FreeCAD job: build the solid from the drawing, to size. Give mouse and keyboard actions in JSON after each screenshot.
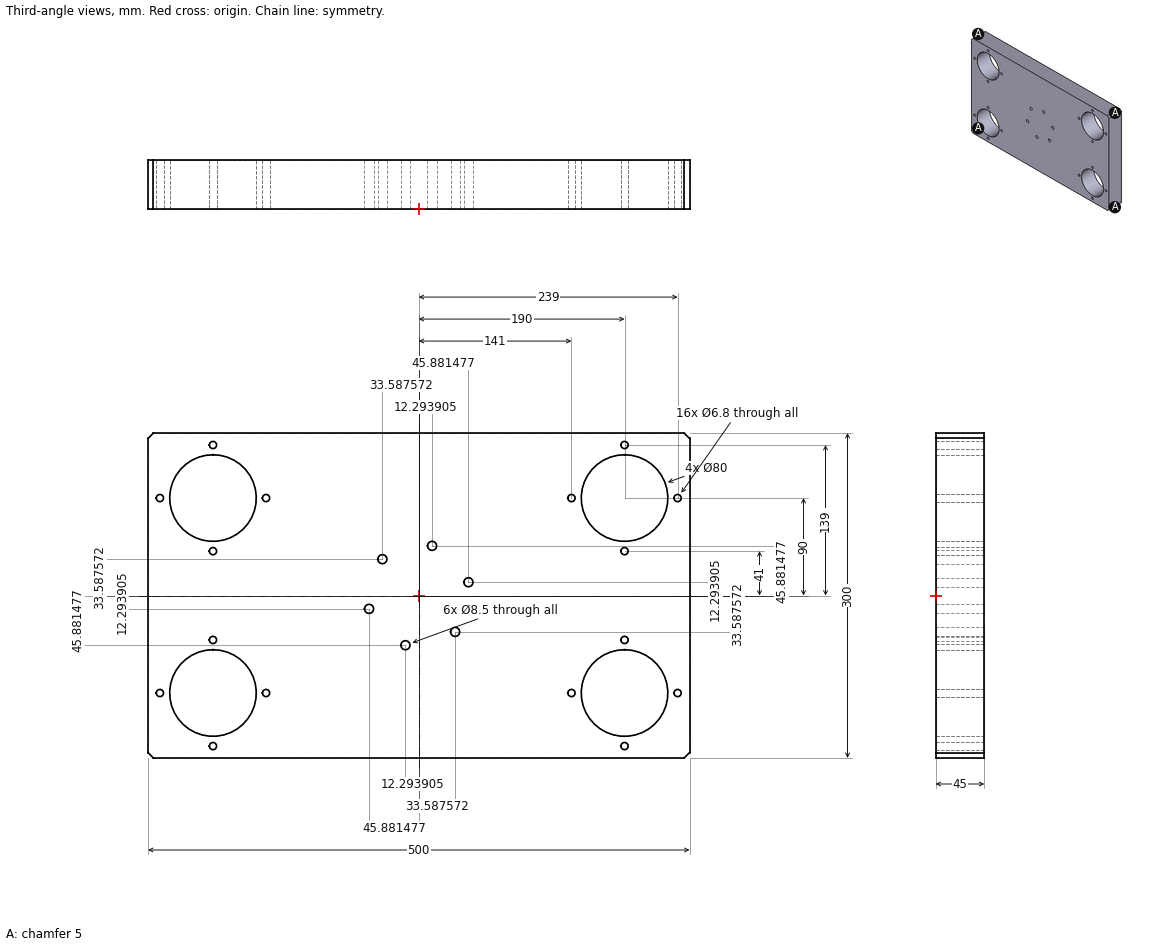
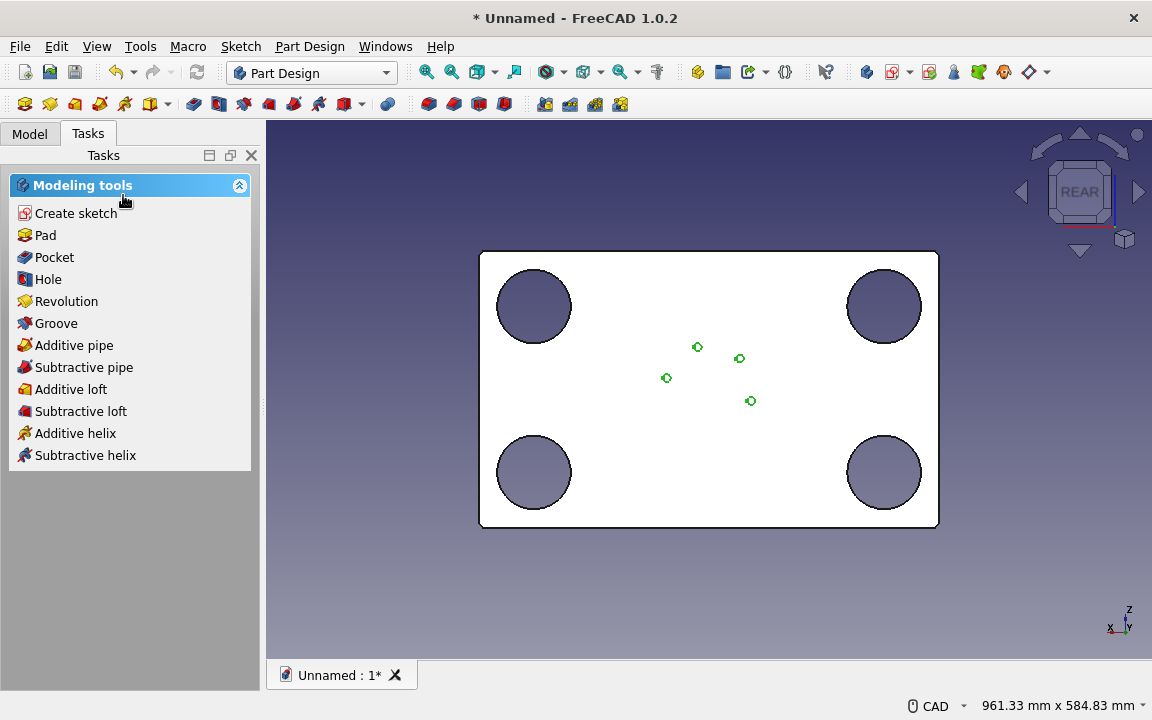
{"action": "left_click", "coordinate": [219, 104]}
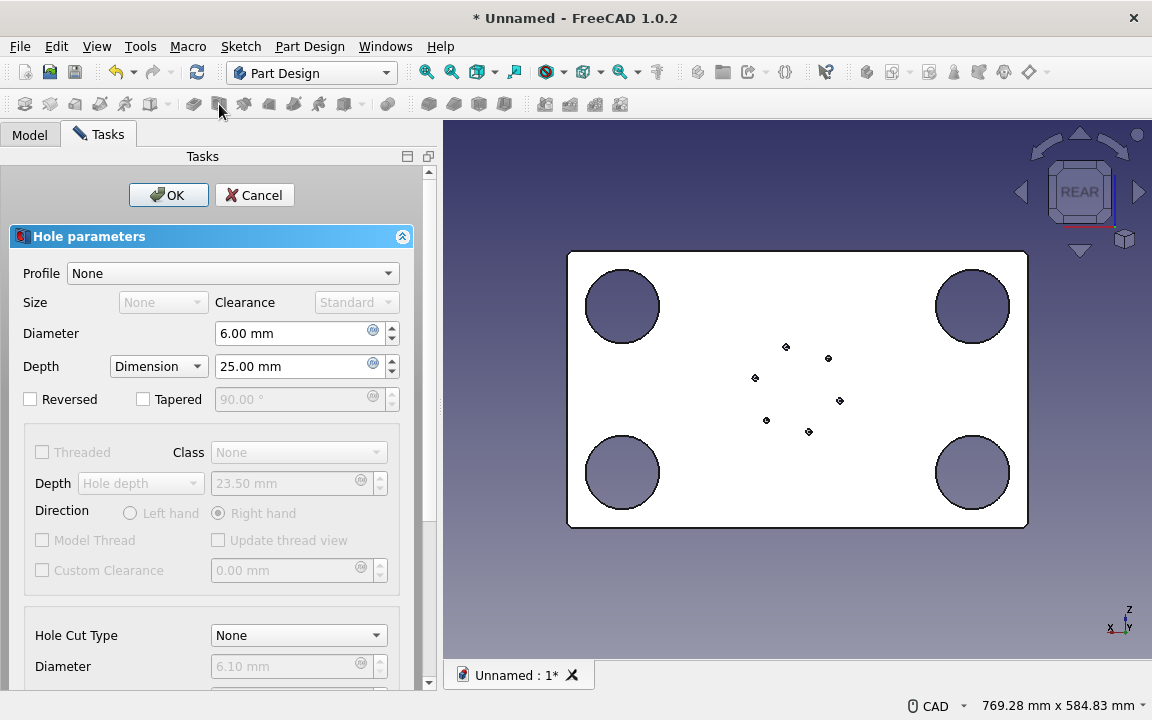
{"action": "triple_click", "coordinate": [300, 334]}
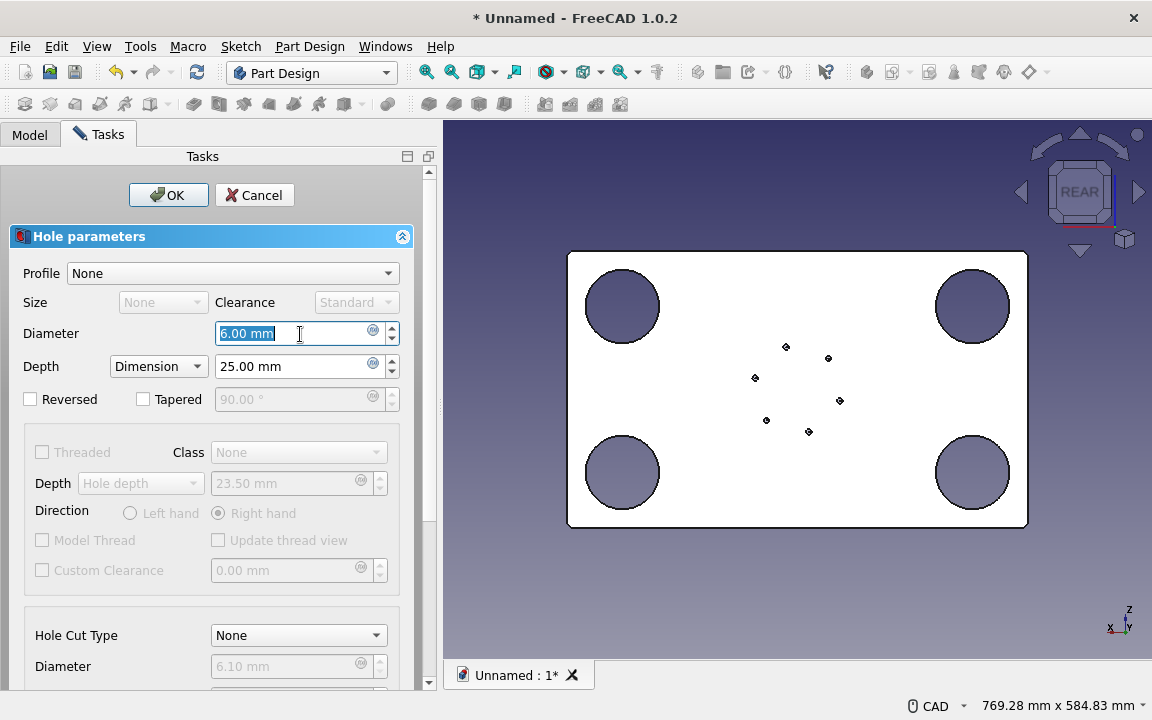
{"action": "type", "text": "8.5"}
{"action": "key", "text": "Tab"}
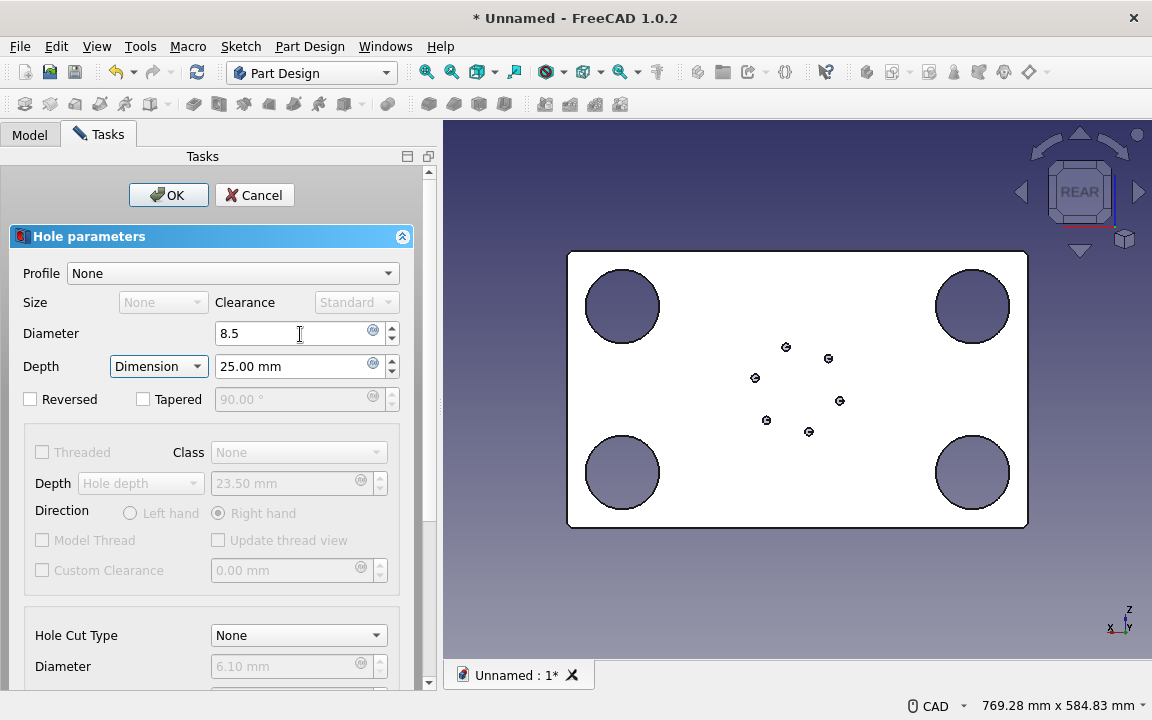
{"action": "left_click", "coordinate": [160, 366]}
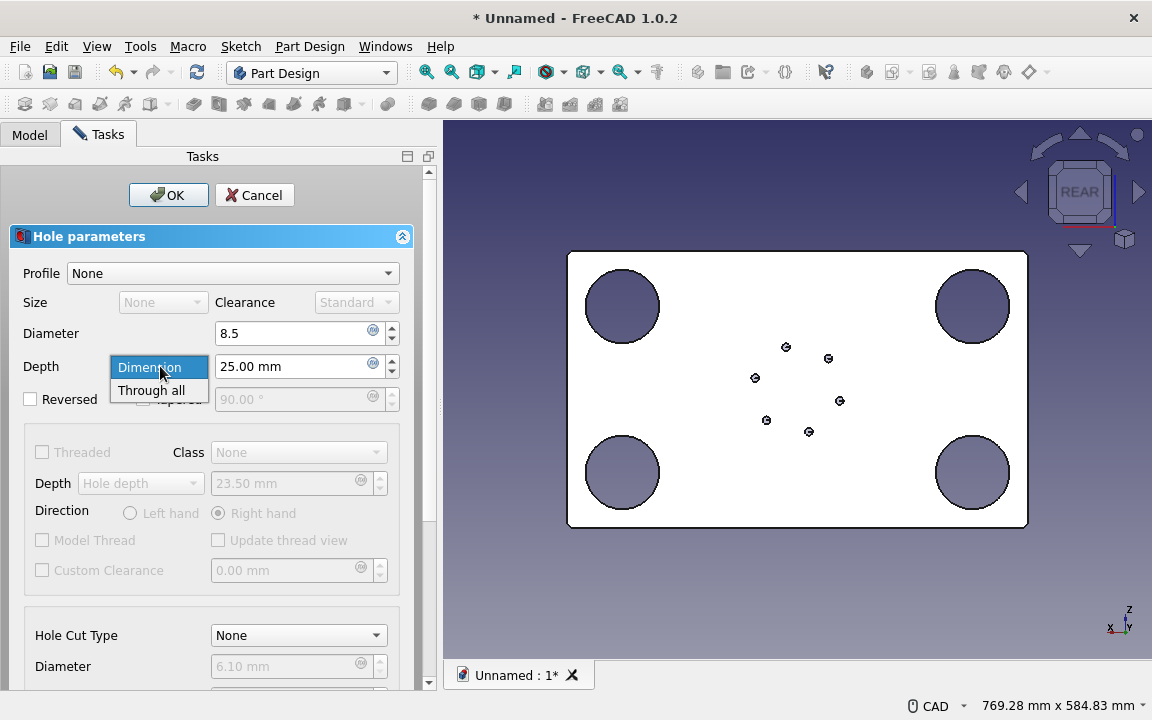
{"action": "left_click", "coordinate": [158, 390]}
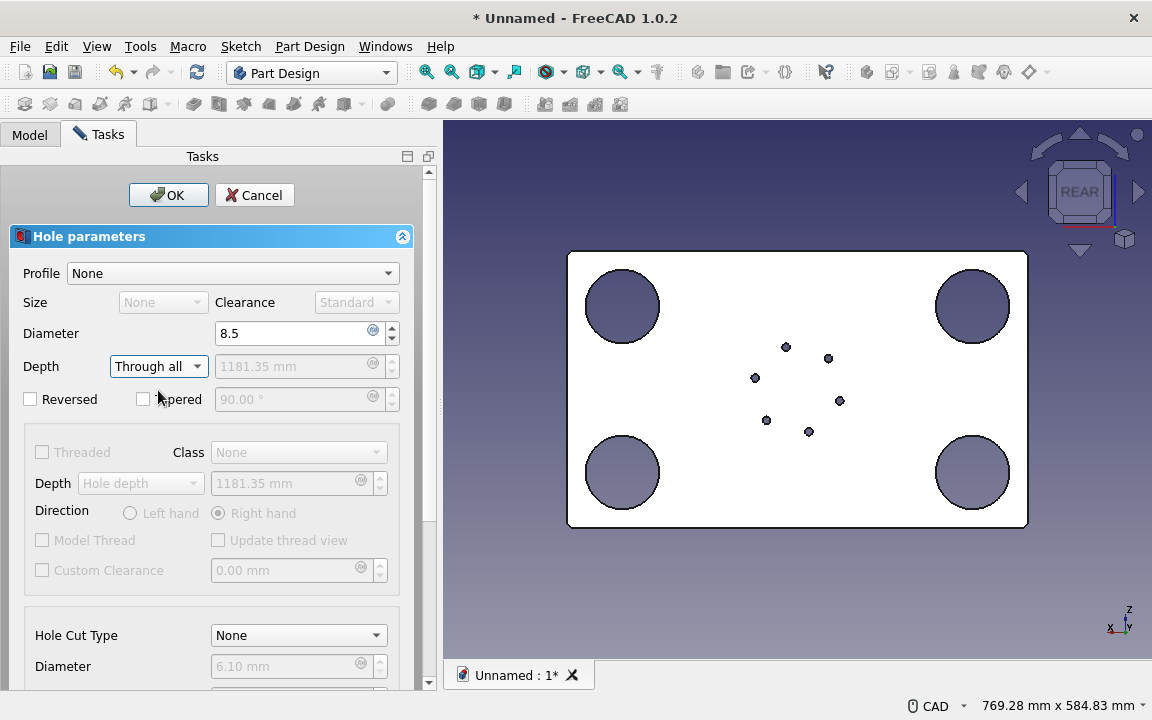
{"action": "left_click", "coordinate": [169, 195]}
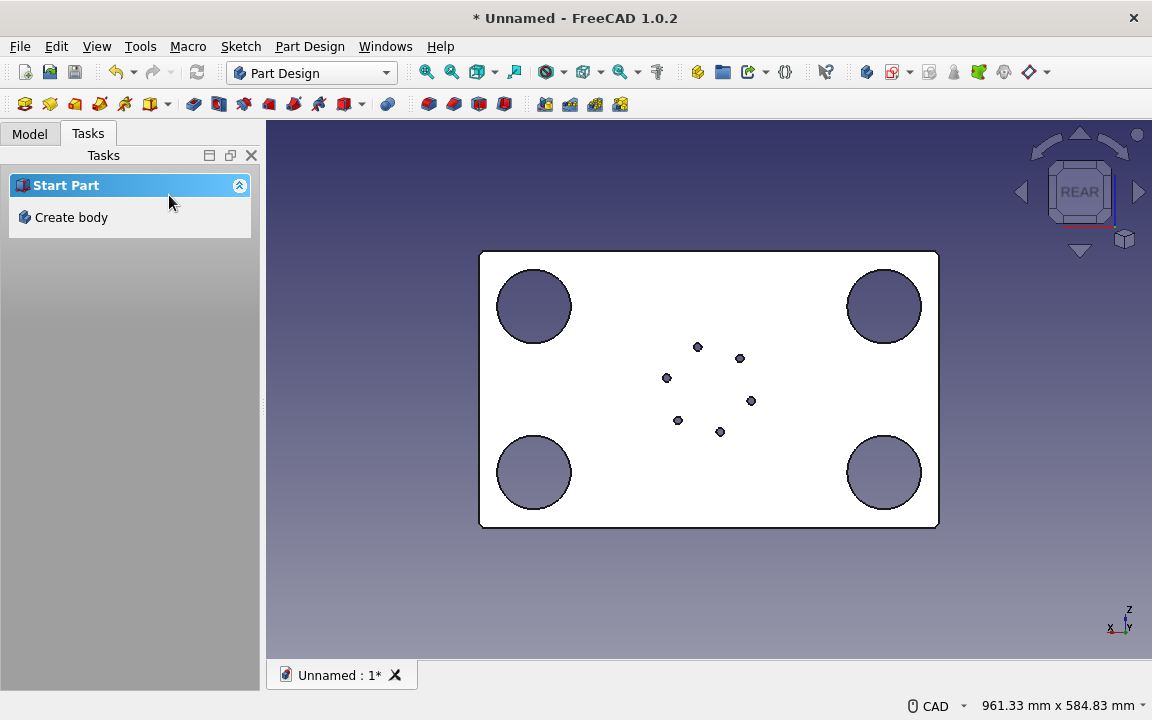
{"action": "left_click", "coordinate": [643, 310]}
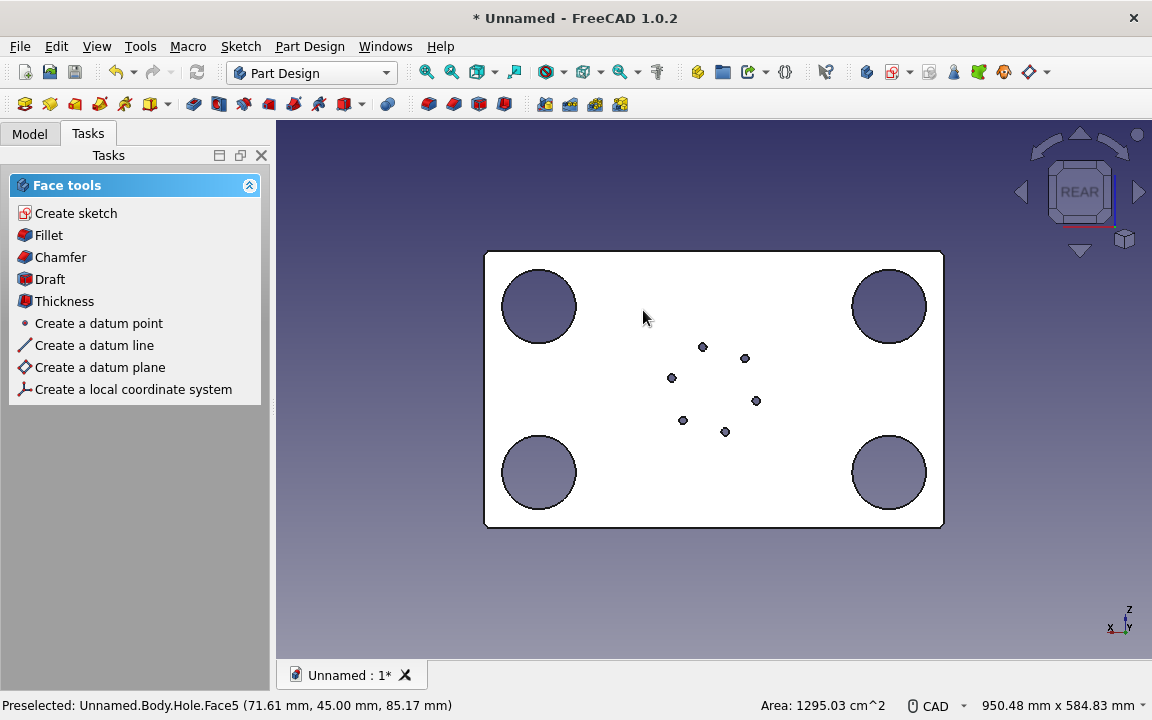
{"action": "left_click", "coordinate": [892, 72]}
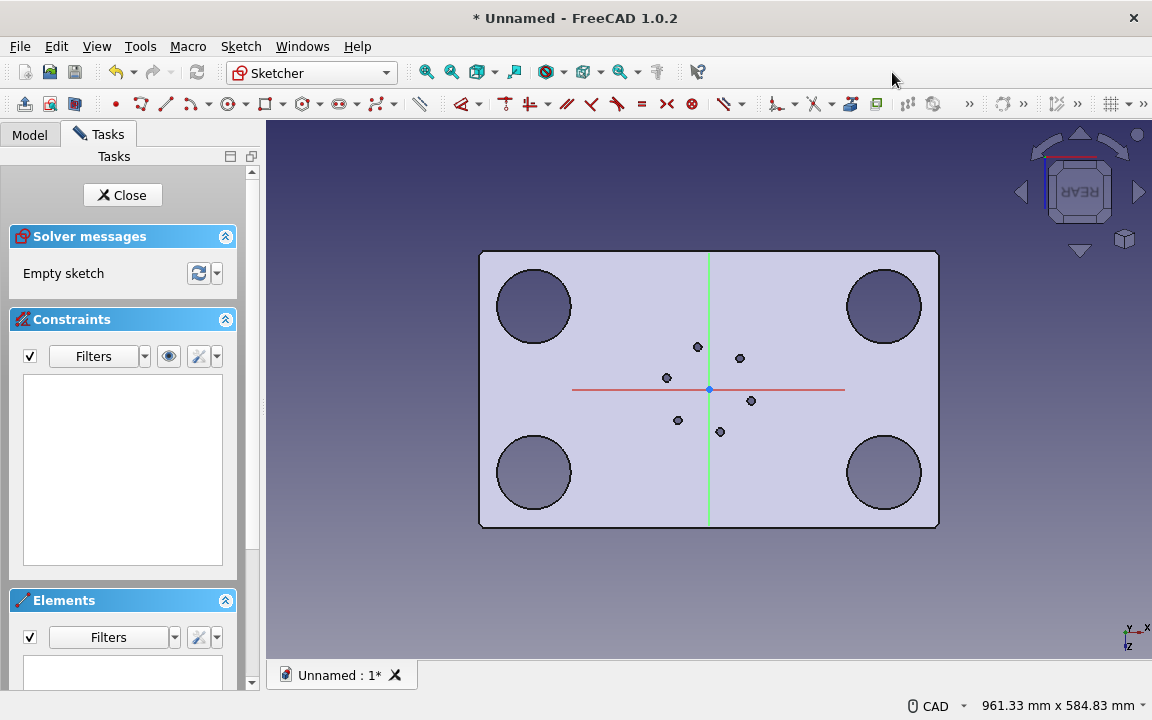
{"action": "left_click", "coordinate": [228, 104]}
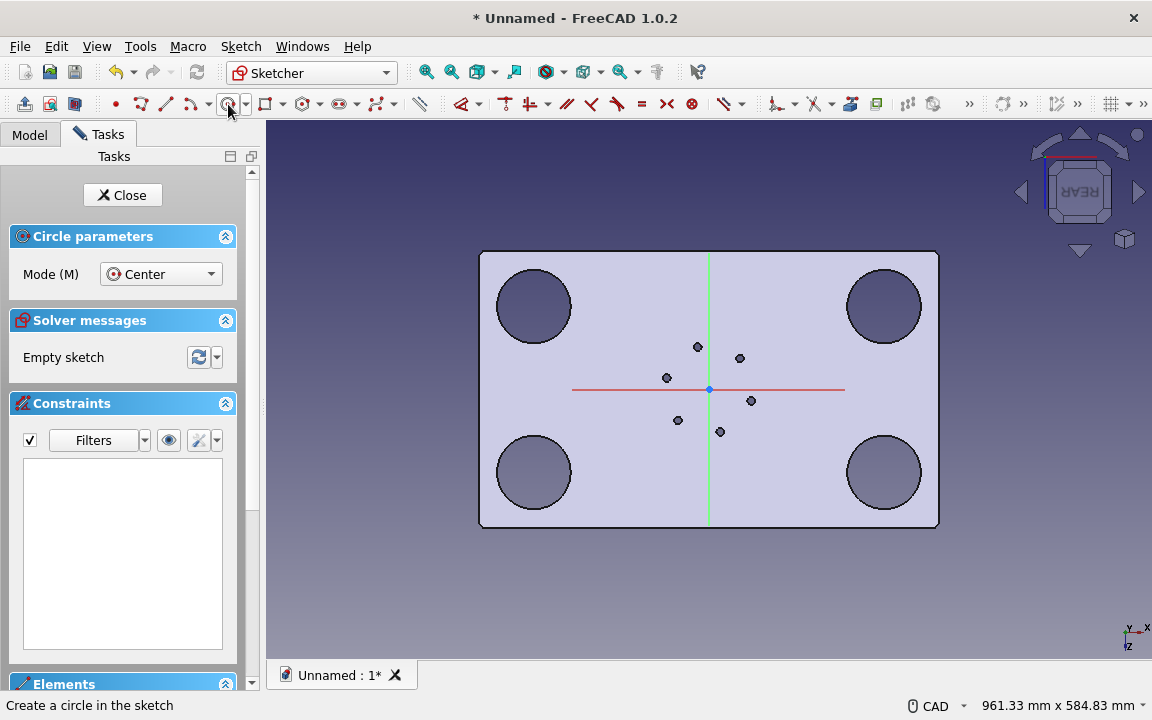
{"action": "scroll", "coordinate": [929, 472], "scroll_direction": "up", "scroll_amount": 10}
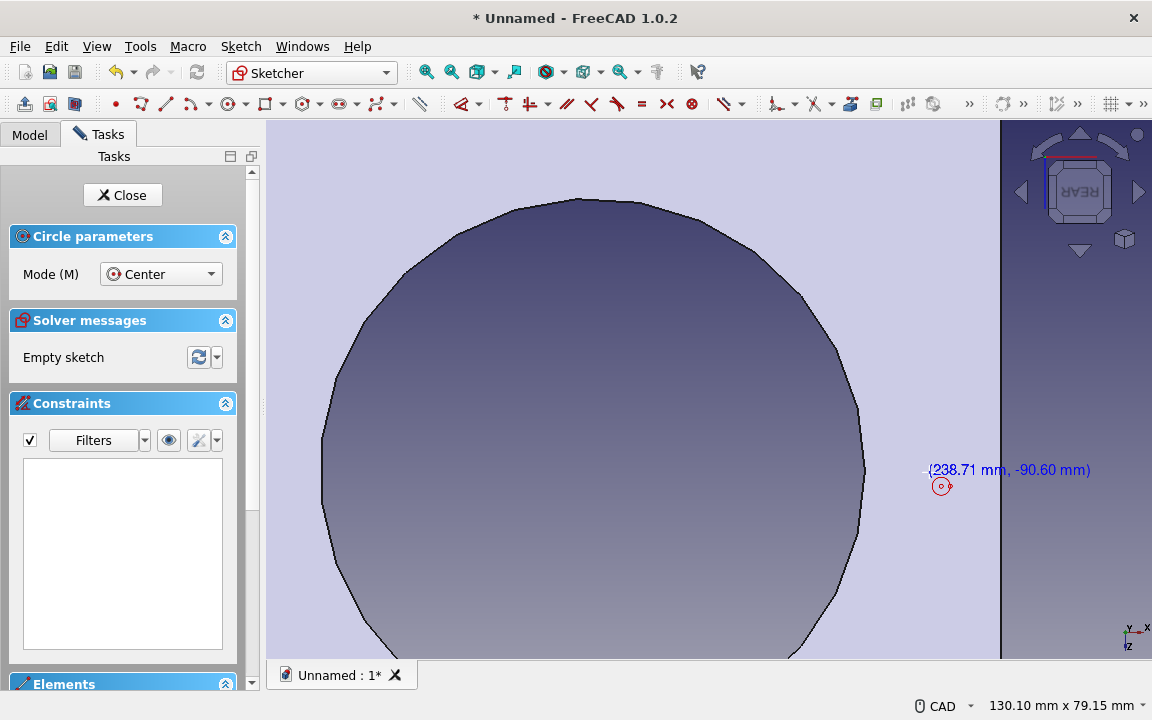
{"action": "scroll", "coordinate": [851, 473], "scroll_direction": "down", "scroll_amount": 10}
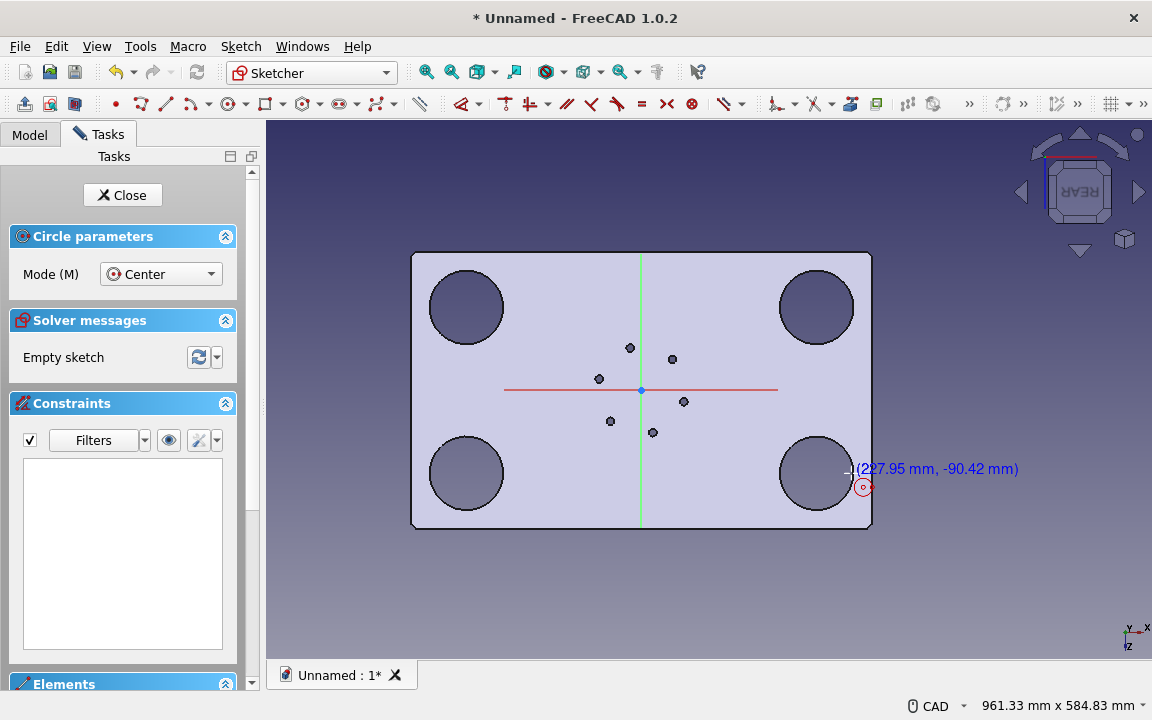
{"action": "left_click", "coordinate": [862, 473]}